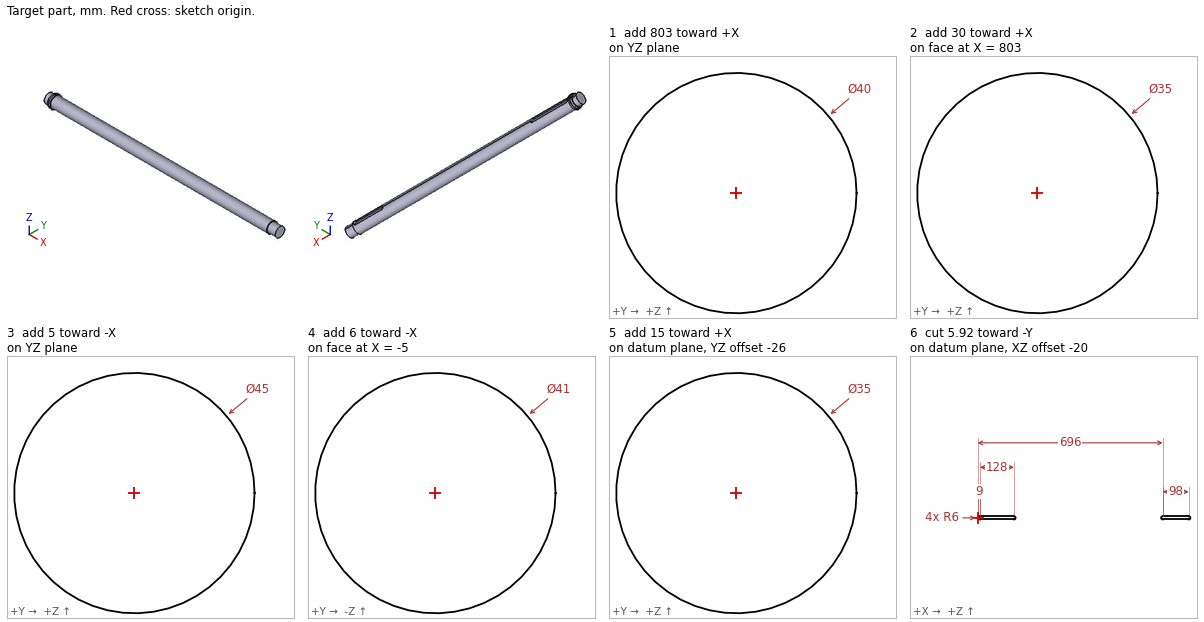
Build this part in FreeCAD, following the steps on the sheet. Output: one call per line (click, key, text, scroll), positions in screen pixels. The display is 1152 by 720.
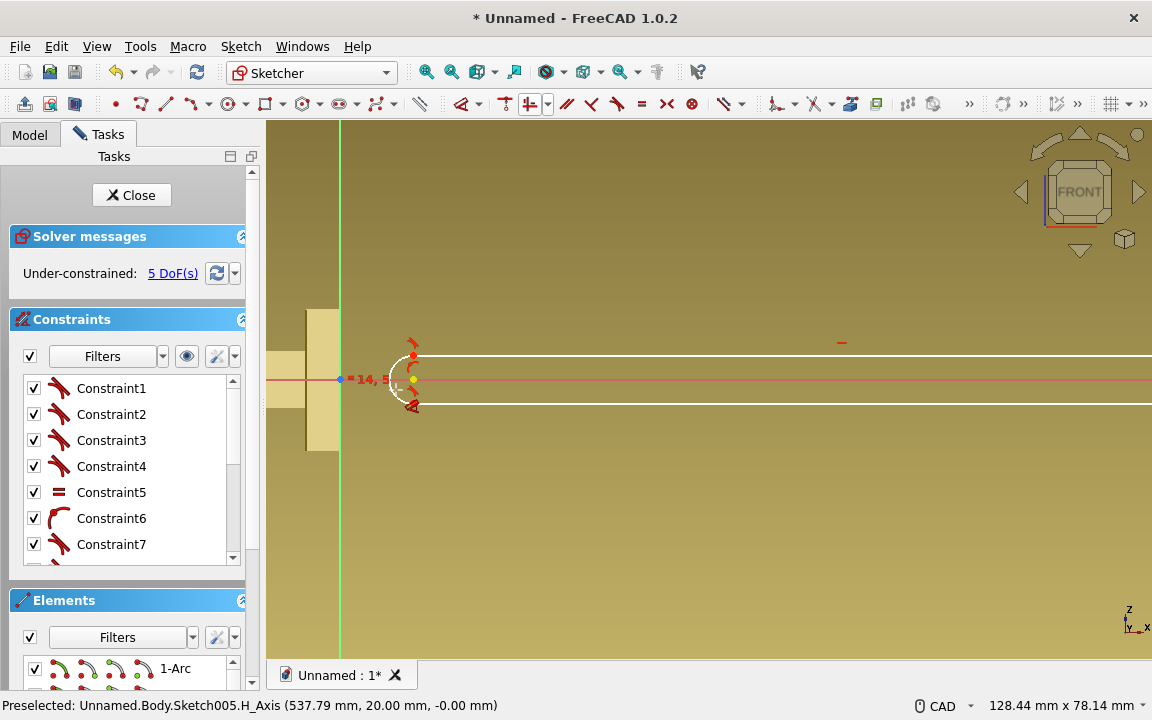
click(389, 380)
click(364, 353)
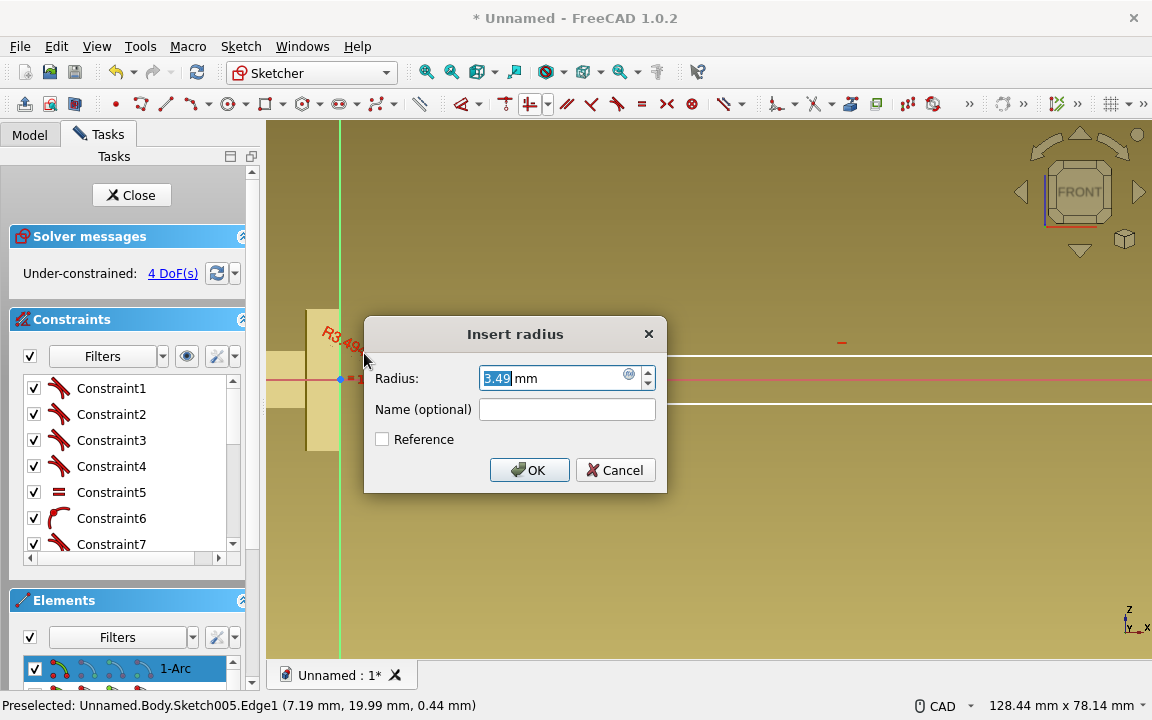
text(6)
key(Return)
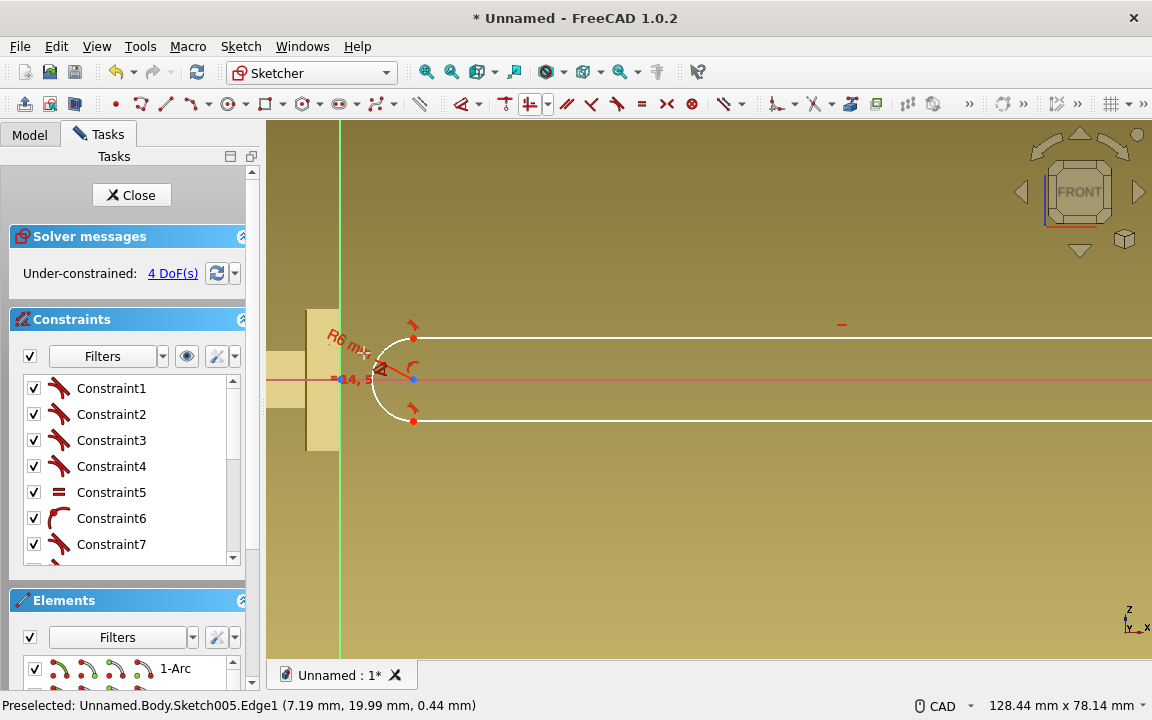
scroll(395, 390, down, 12)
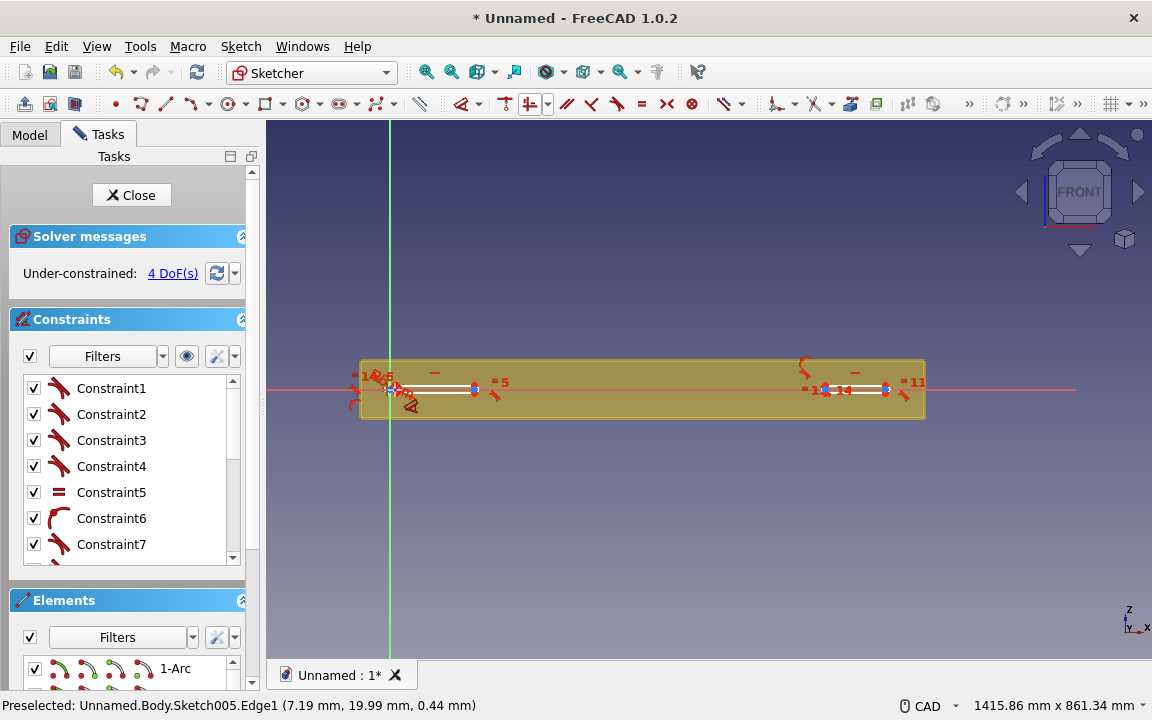
scroll(844, 386, up, 7)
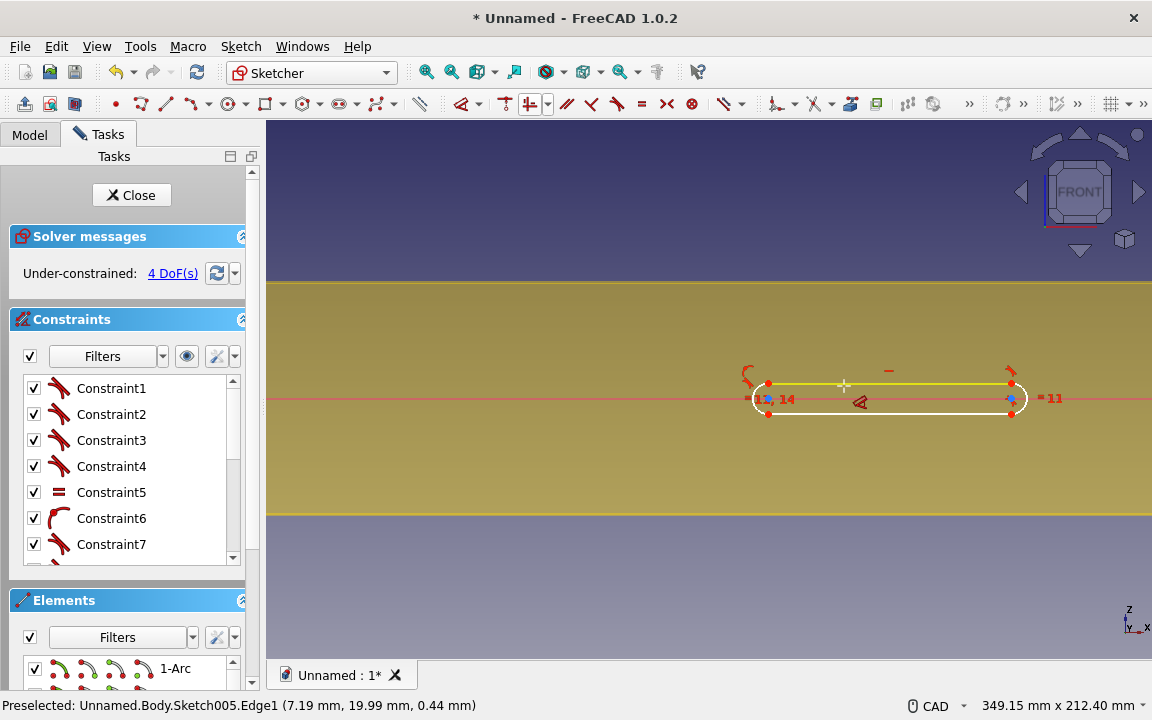
click(841, 384)
click(878, 350)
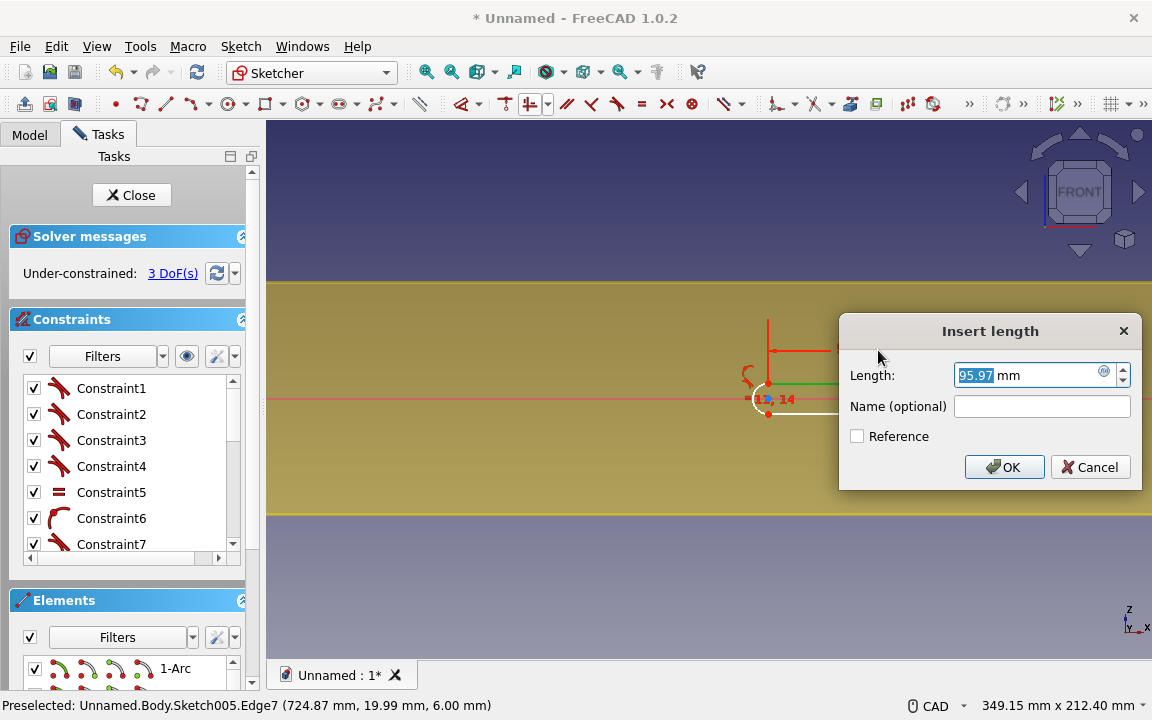
text(98)
key(Return)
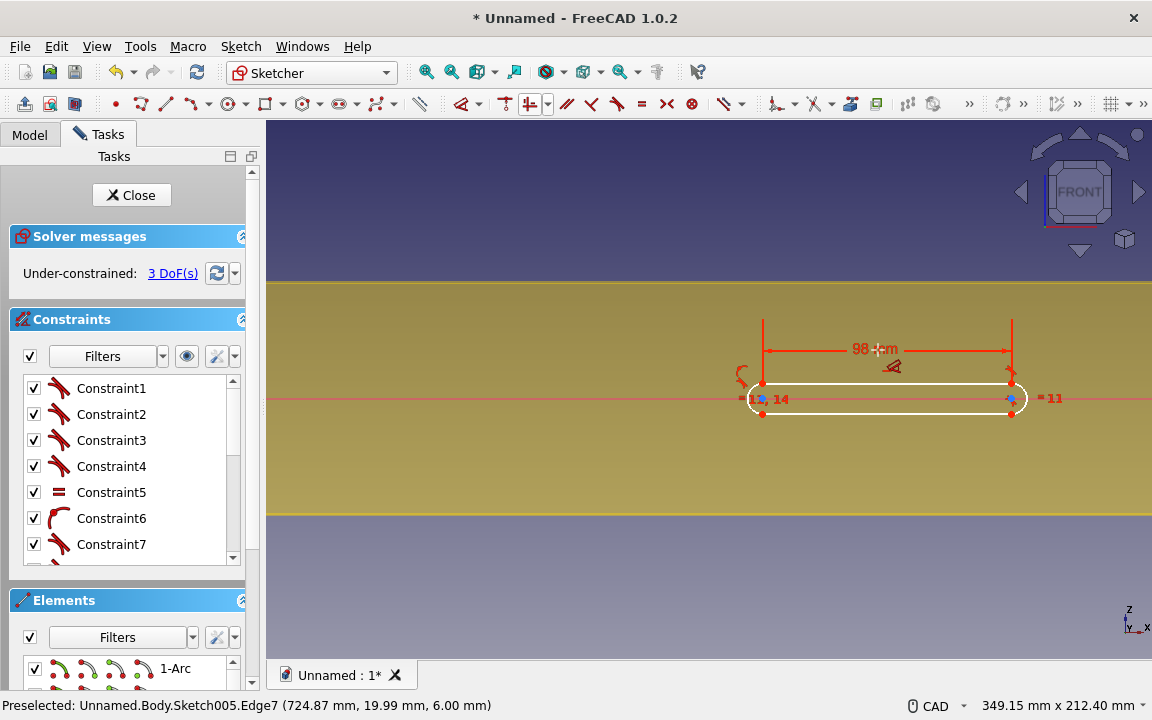
scroll(845, 386, down, 7)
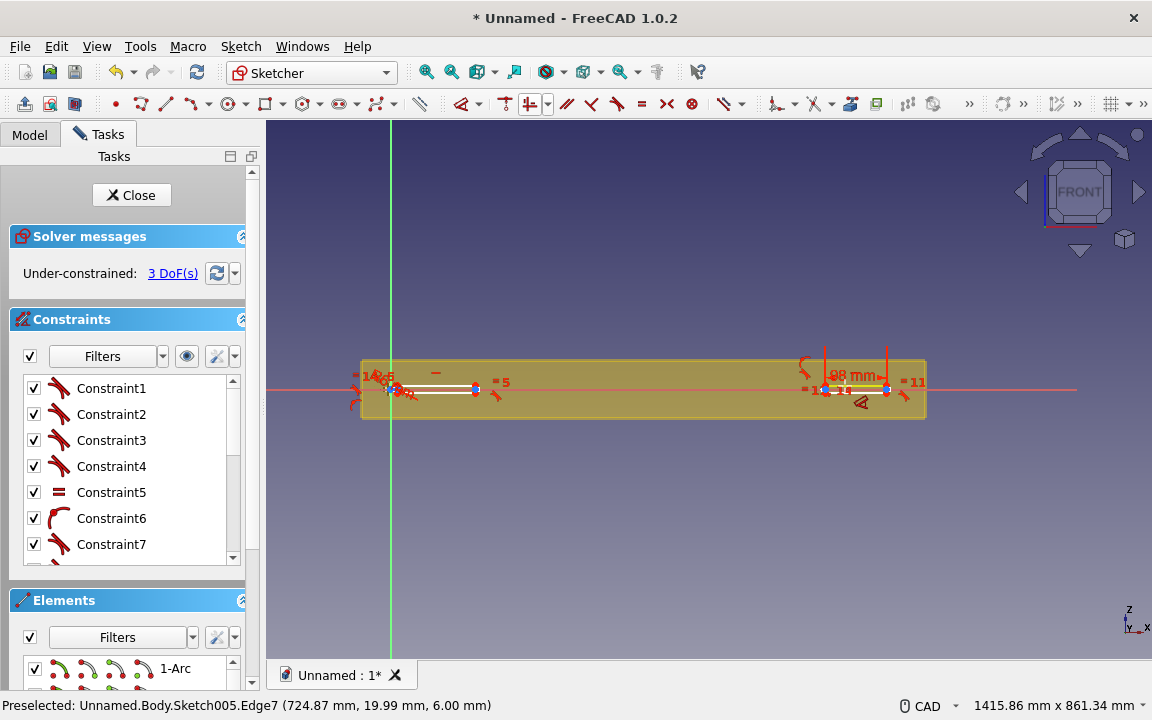
scroll(398, 386, up, 10)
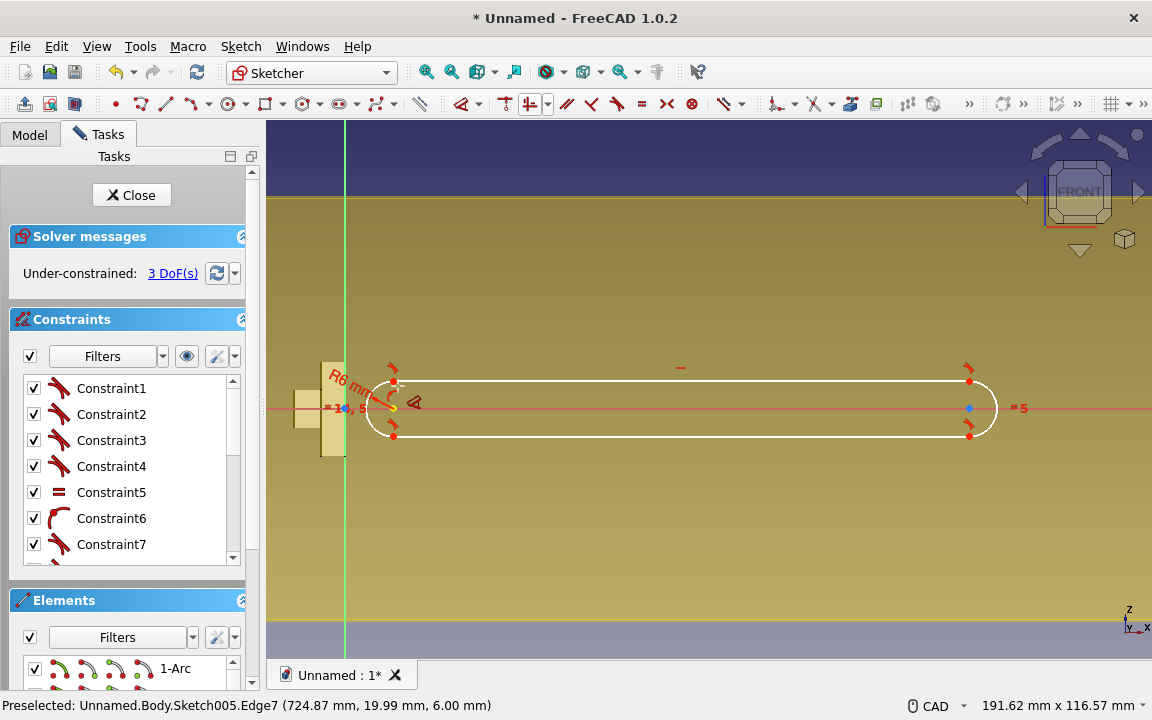
click(394, 381)
click(369, 347)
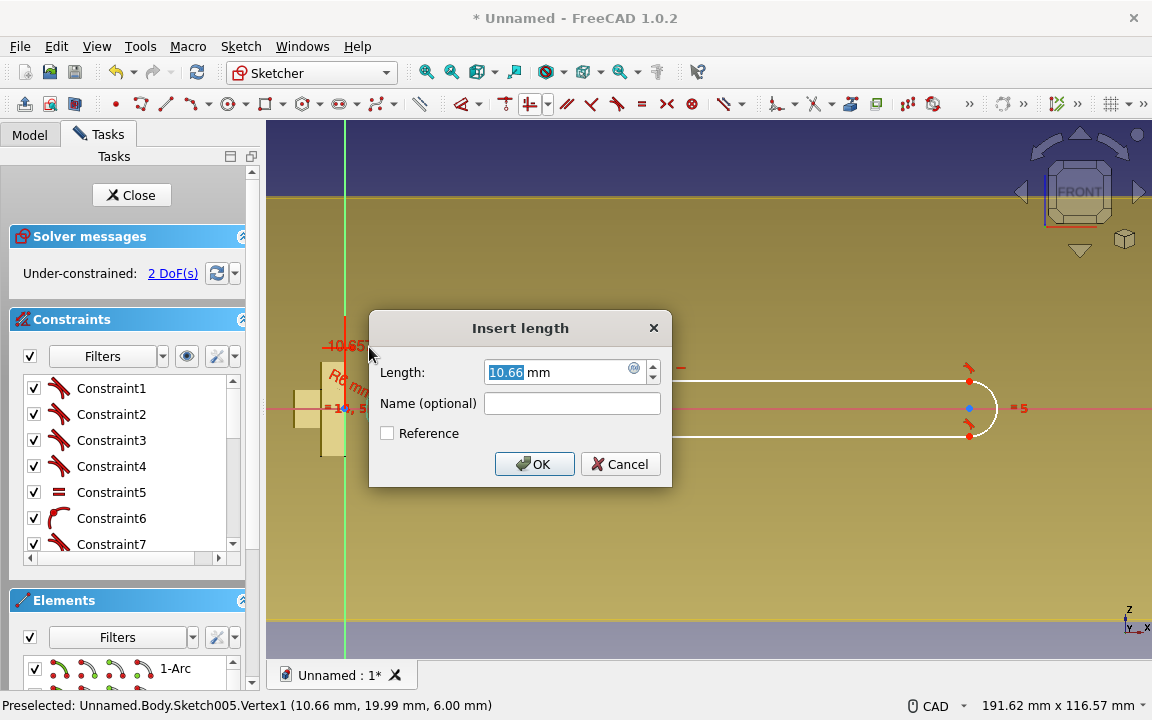
text(9)
key(Return)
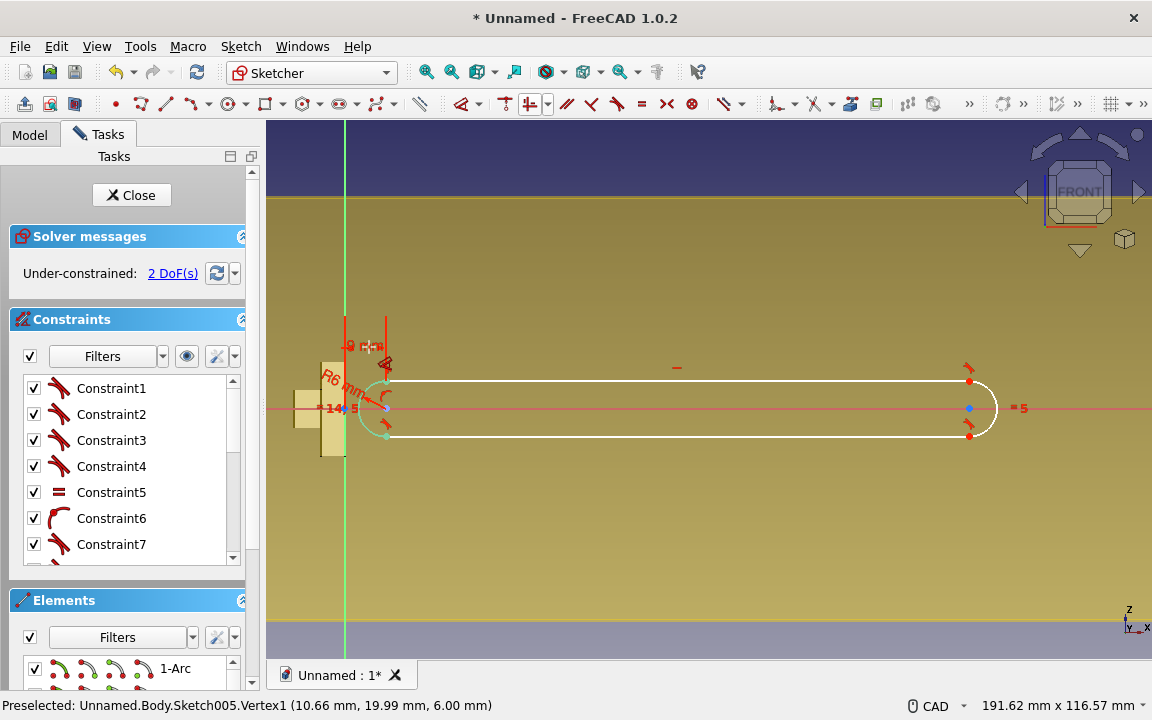
click(561, 381)
click(678, 347)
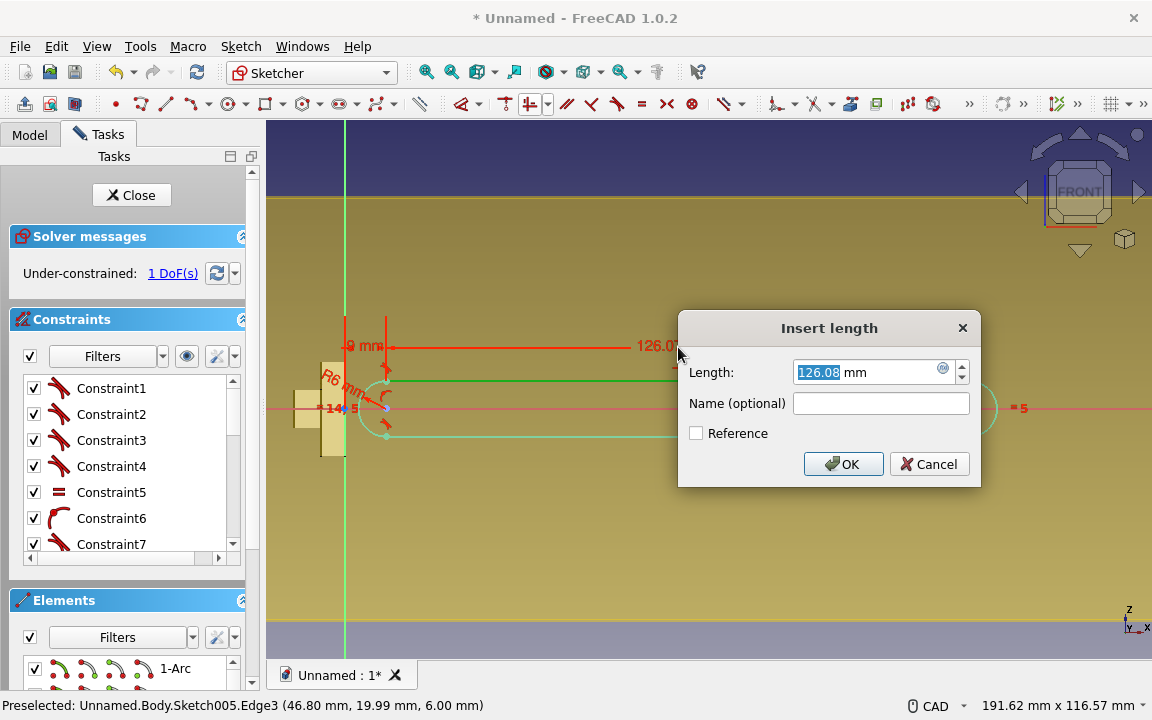
text(128)
key(Return)